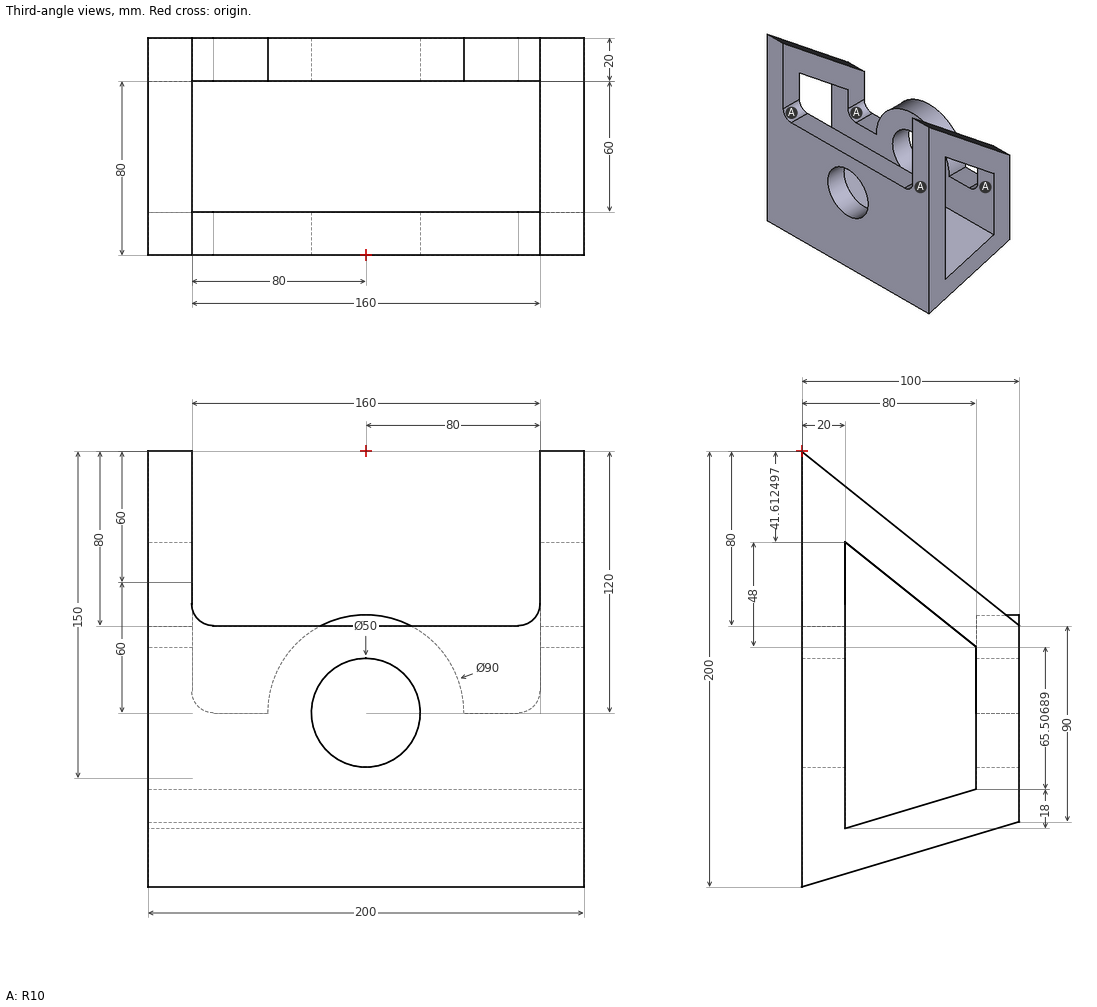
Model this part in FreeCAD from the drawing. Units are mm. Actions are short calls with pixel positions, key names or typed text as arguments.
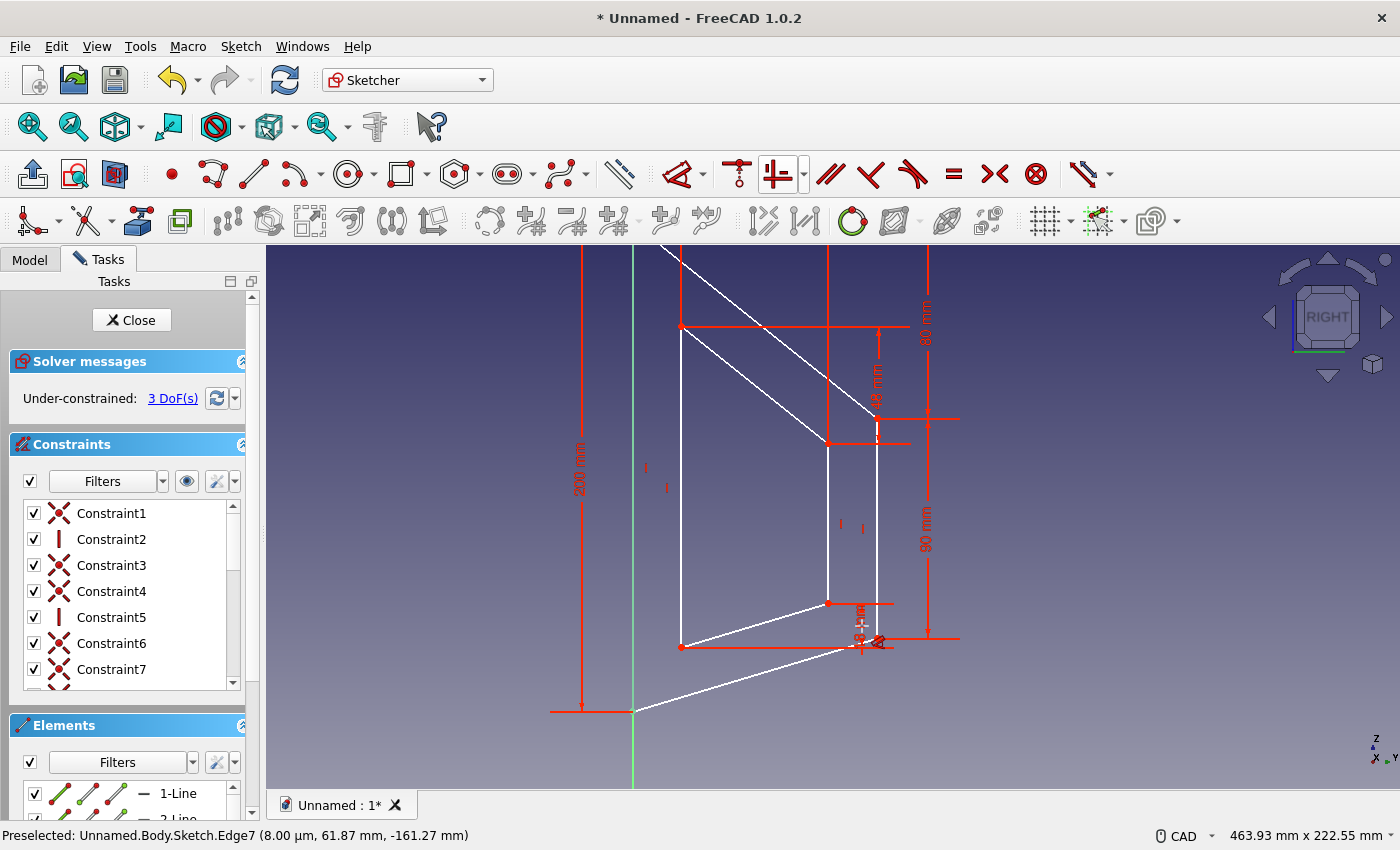
click(877, 639)
click(699, 673)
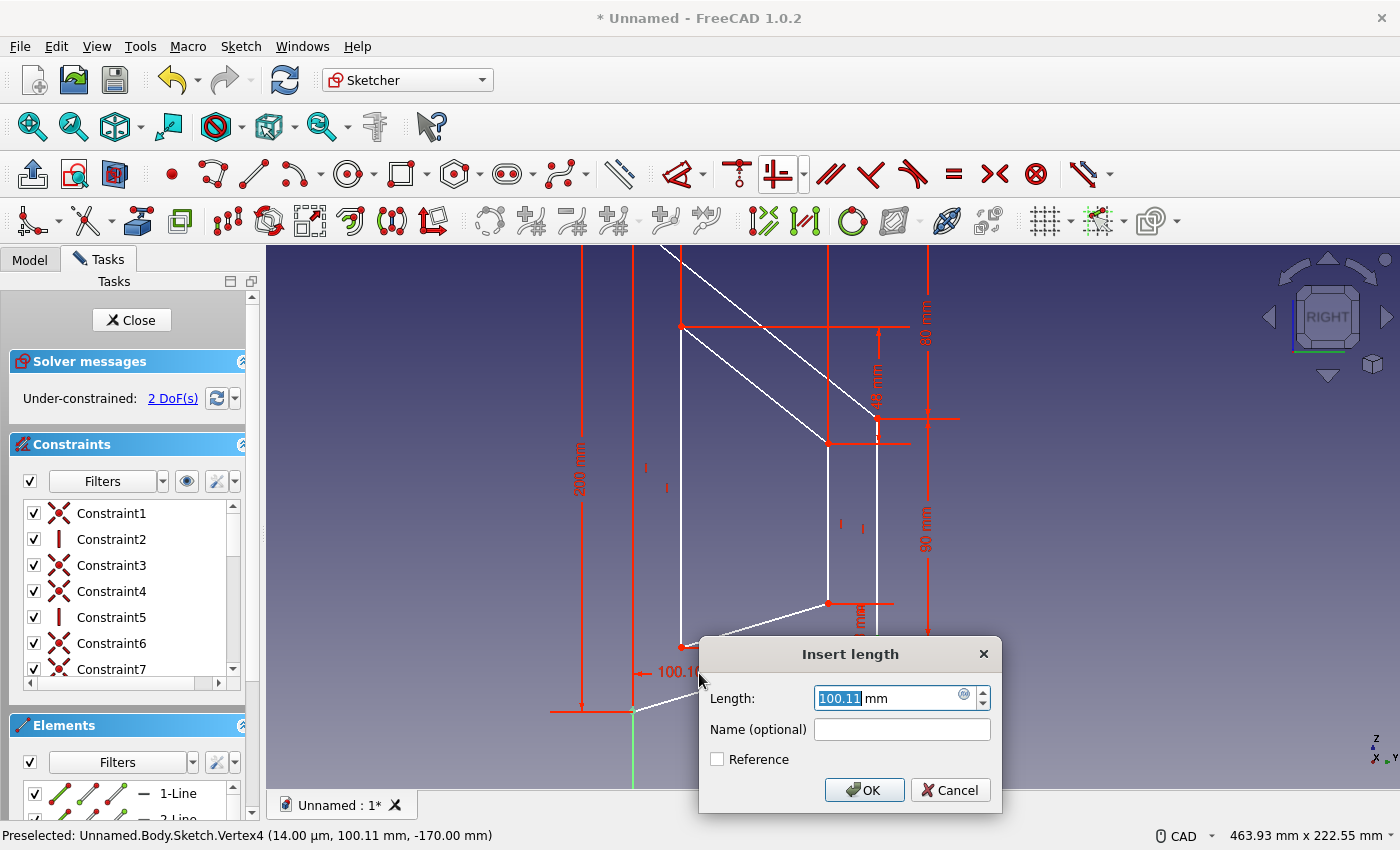
text(100)
key(Return)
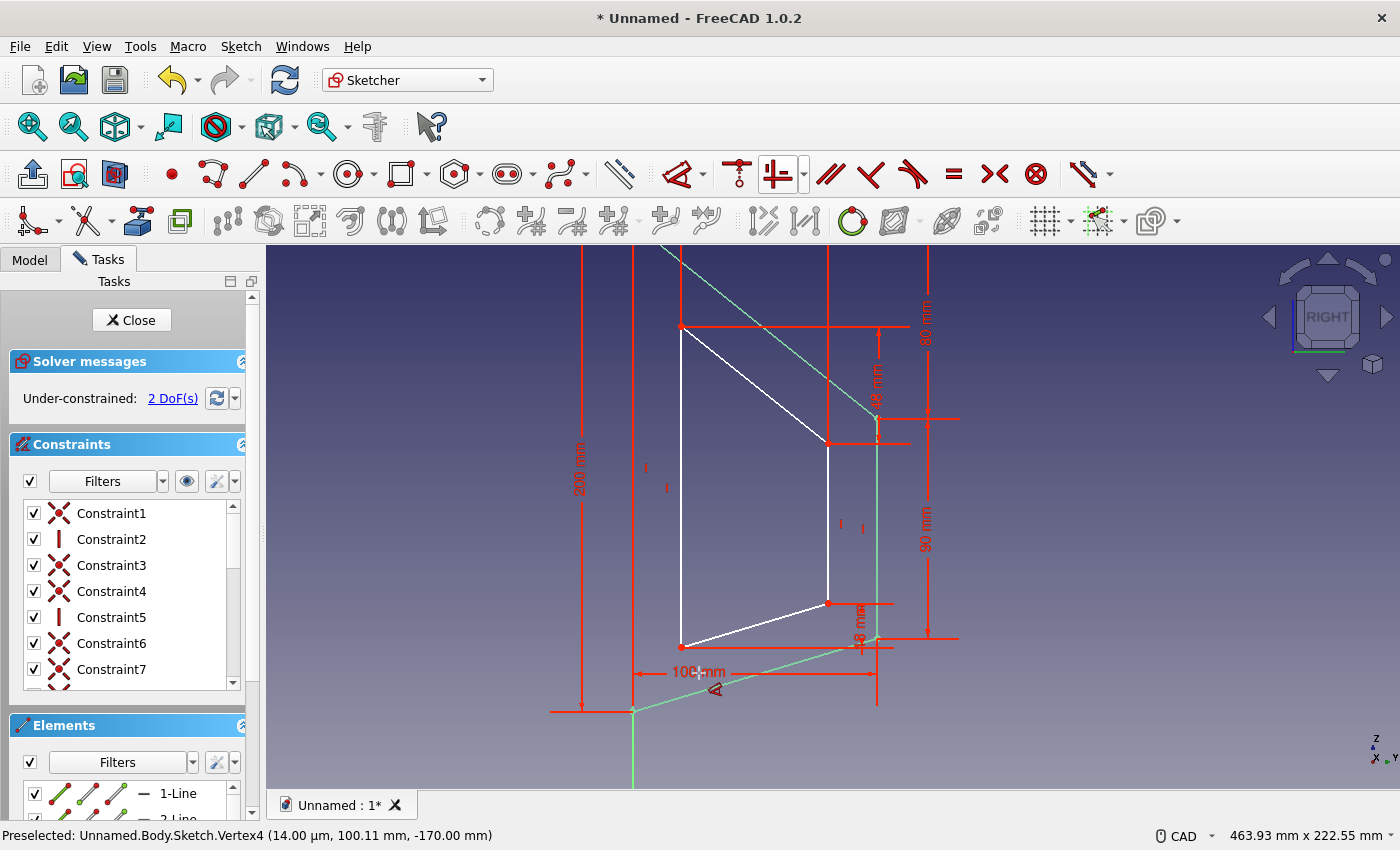
click(828, 492)
click(862, 487)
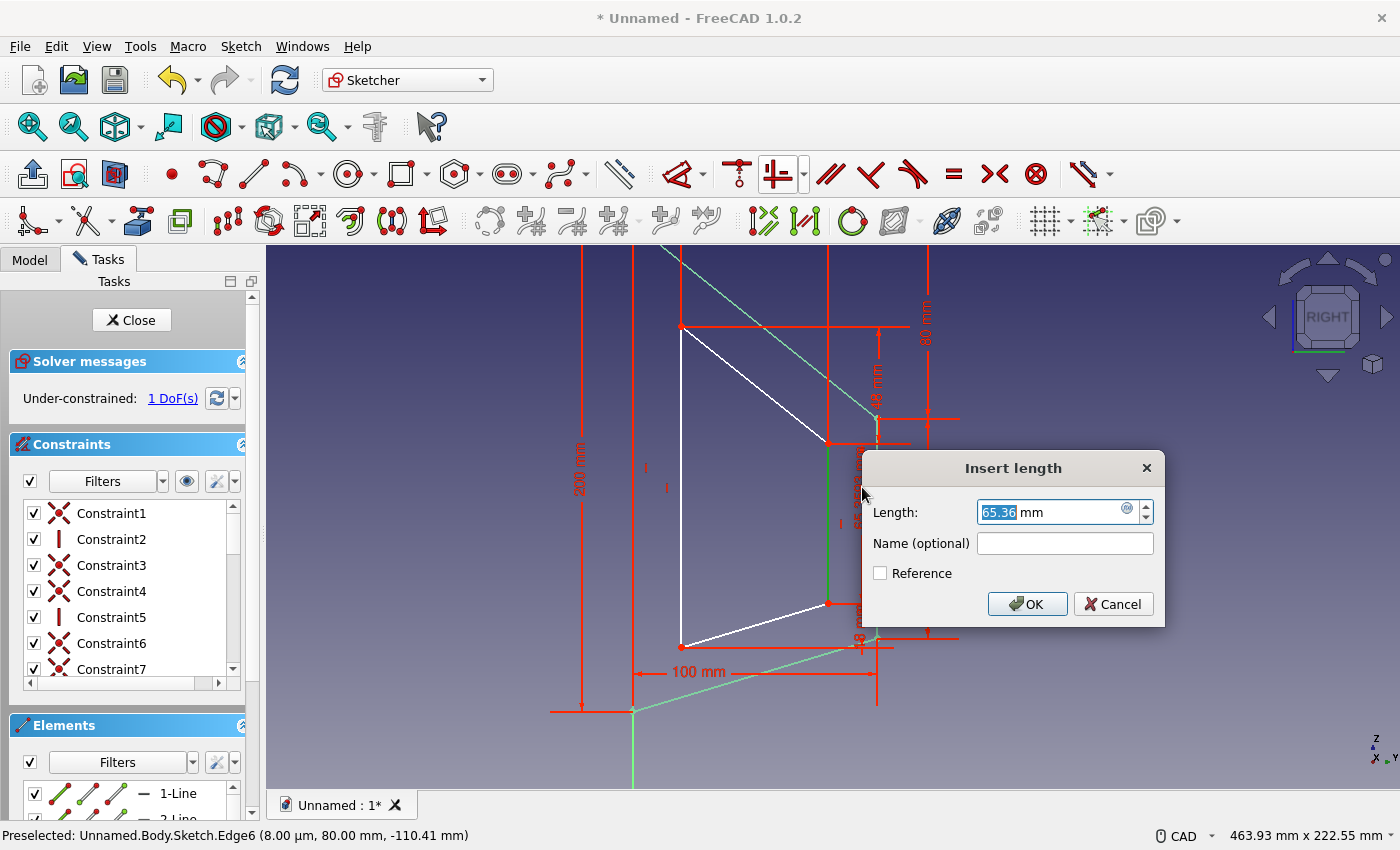
text(65.50689)
key(Return)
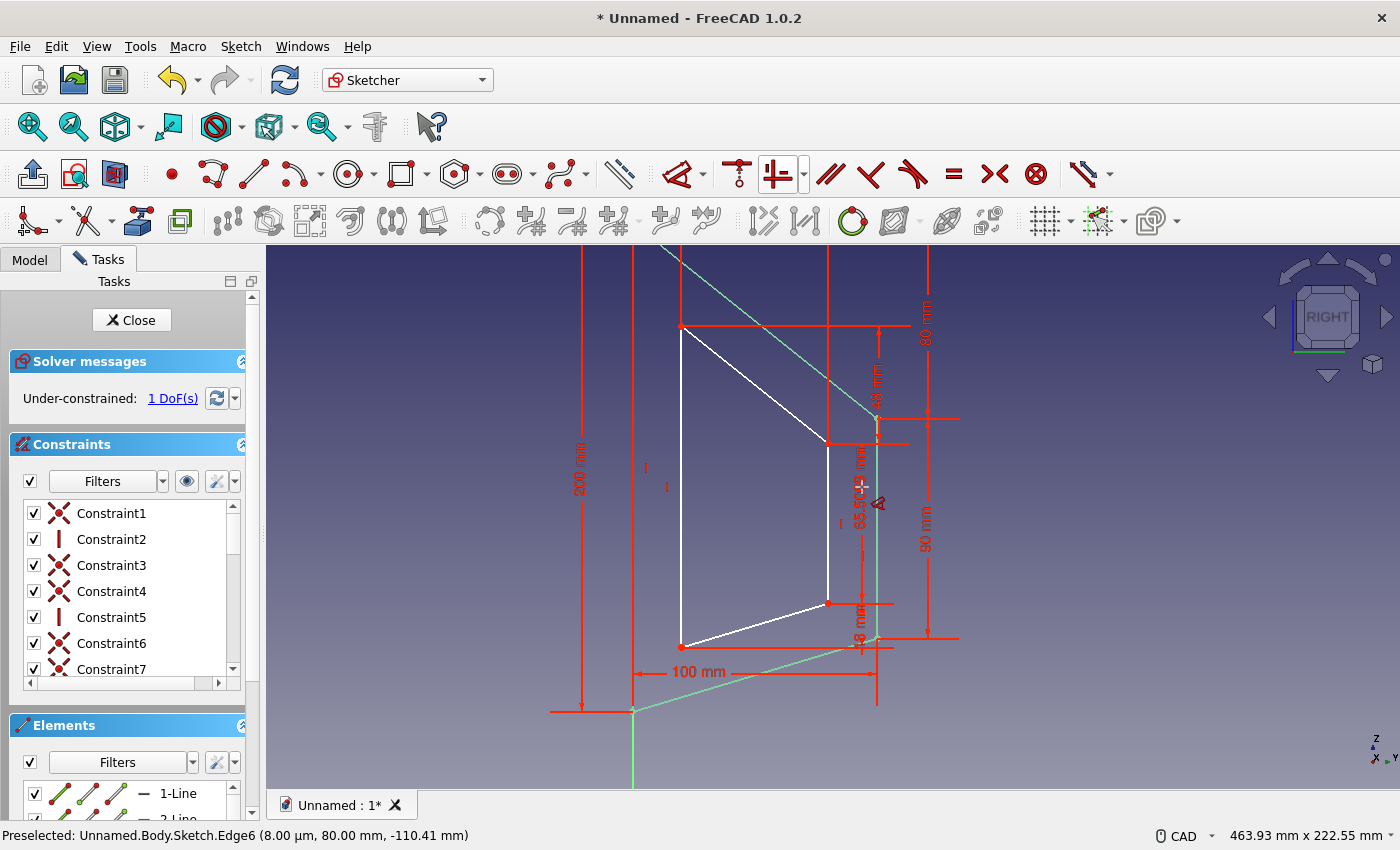
click(681, 326)
click(599, 300)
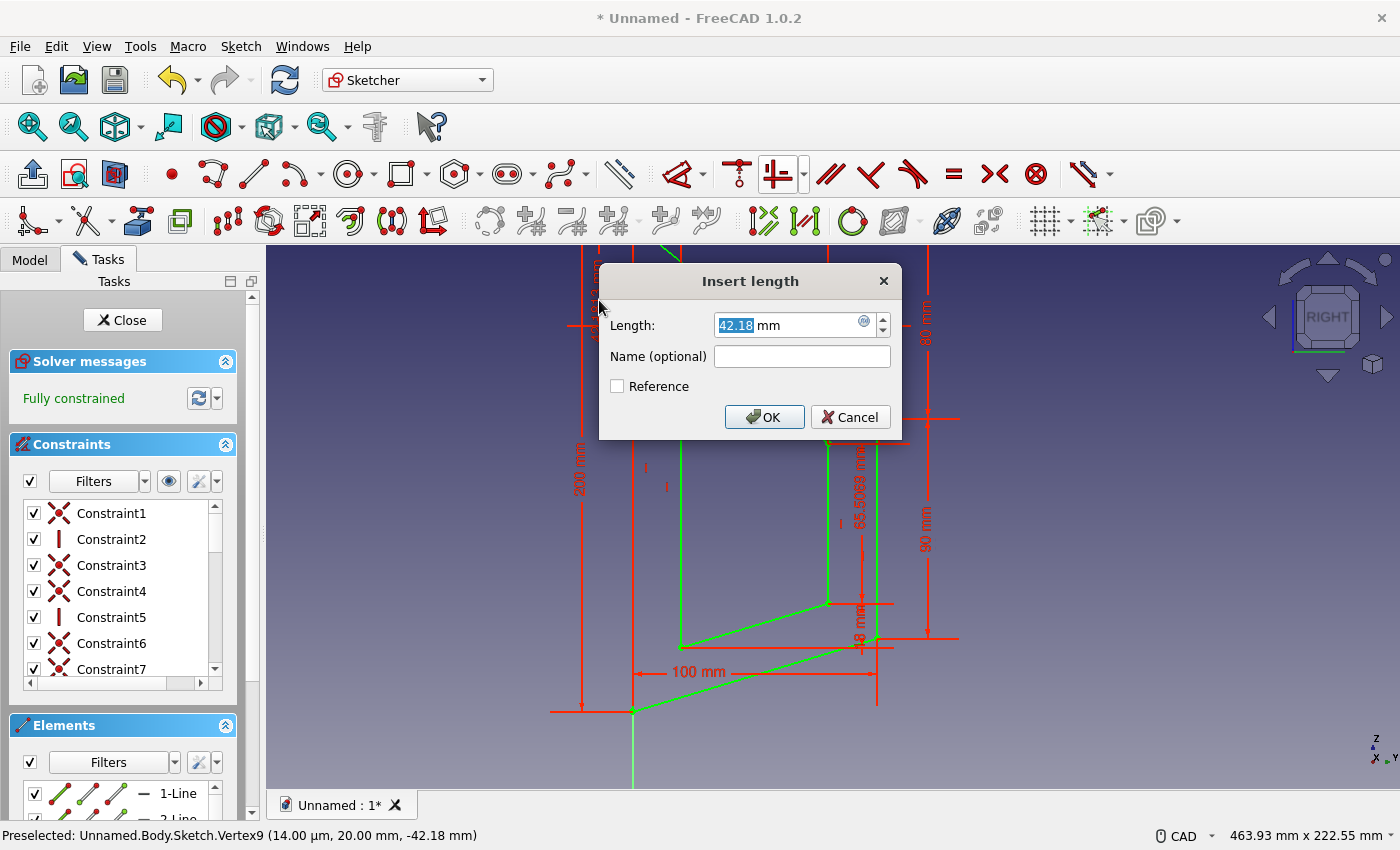
text(41.612497)
key(Return)
key(Escape)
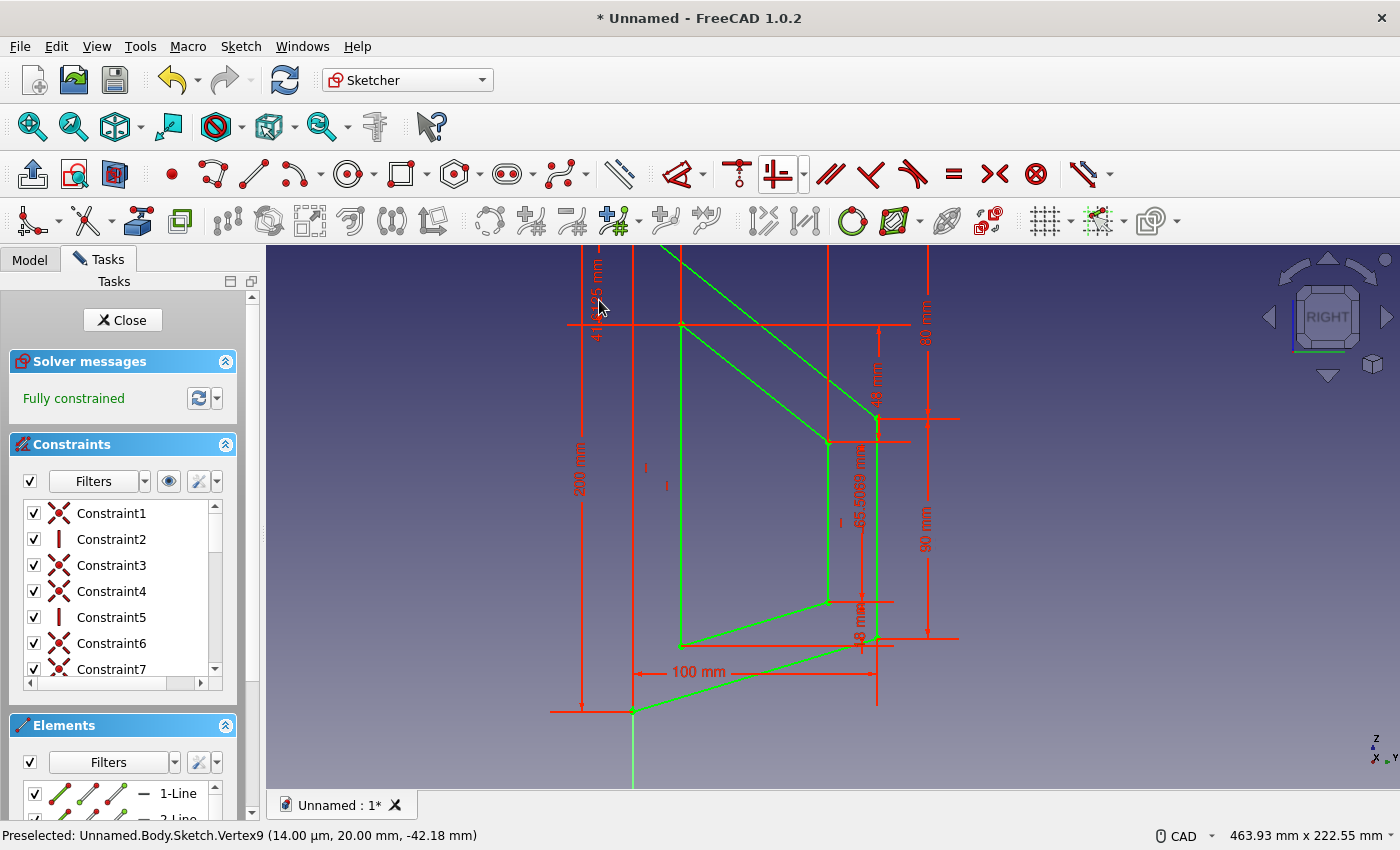
click(123, 320)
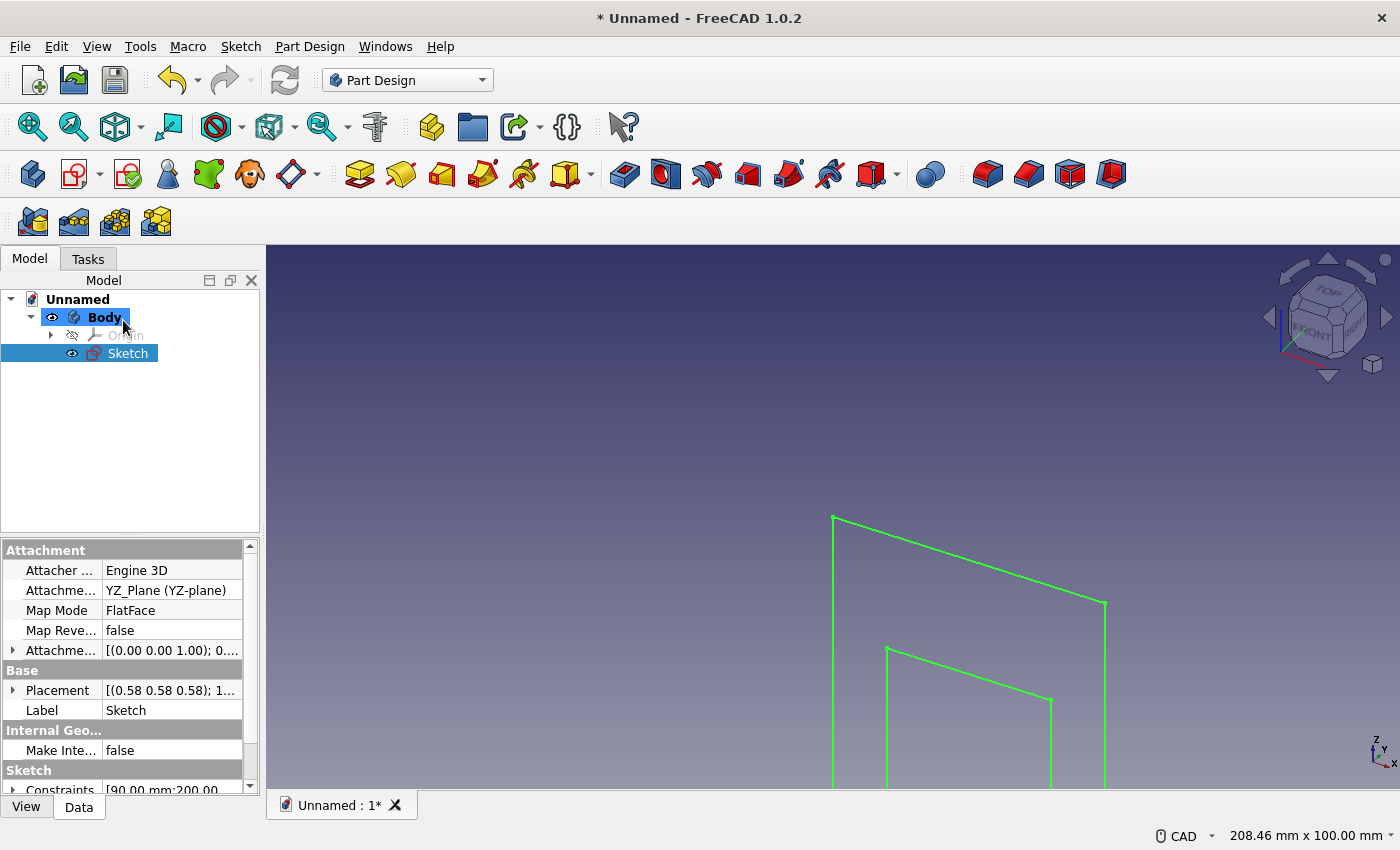
click(360, 174)